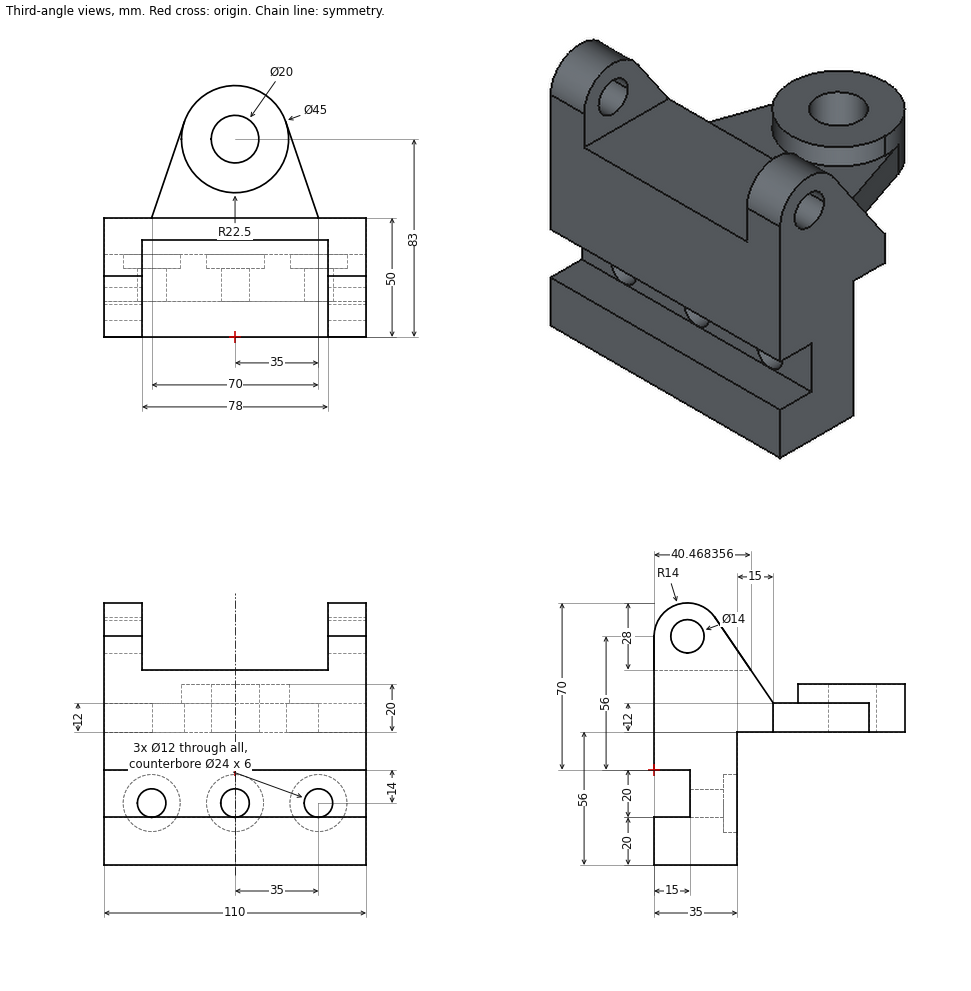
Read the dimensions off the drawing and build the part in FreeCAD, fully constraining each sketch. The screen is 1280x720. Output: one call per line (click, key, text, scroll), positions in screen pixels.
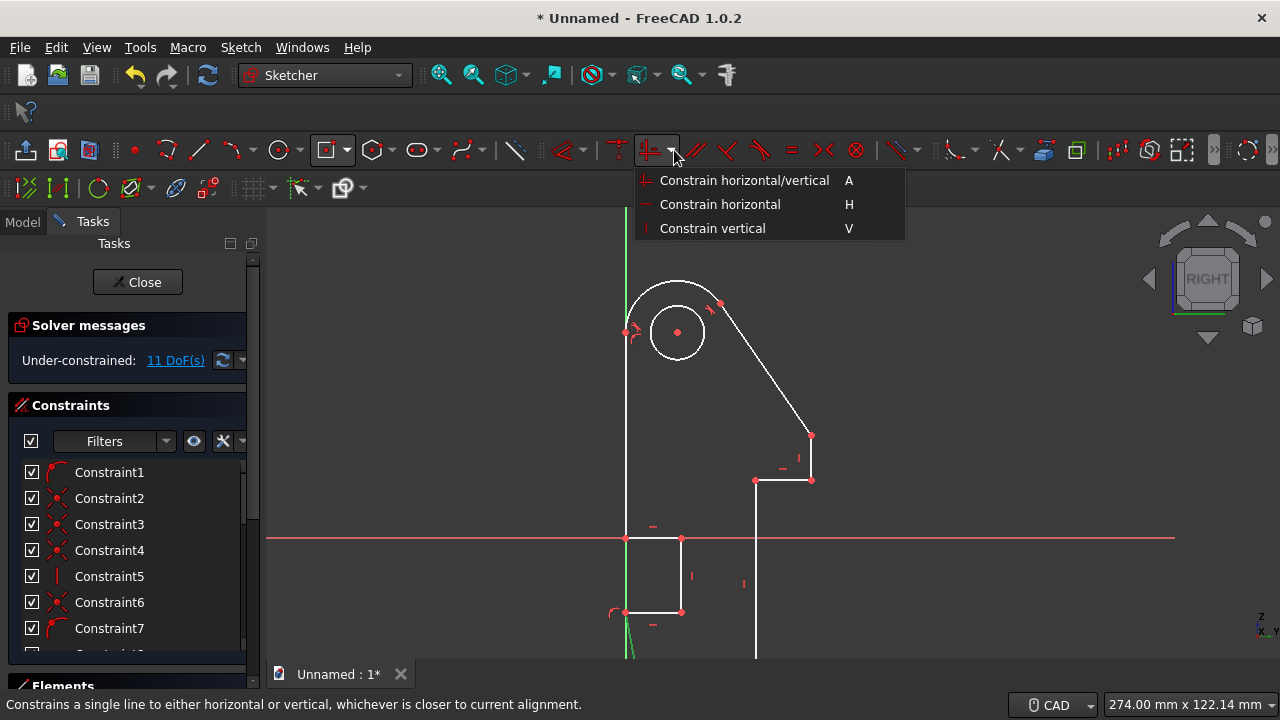
click(770, 228)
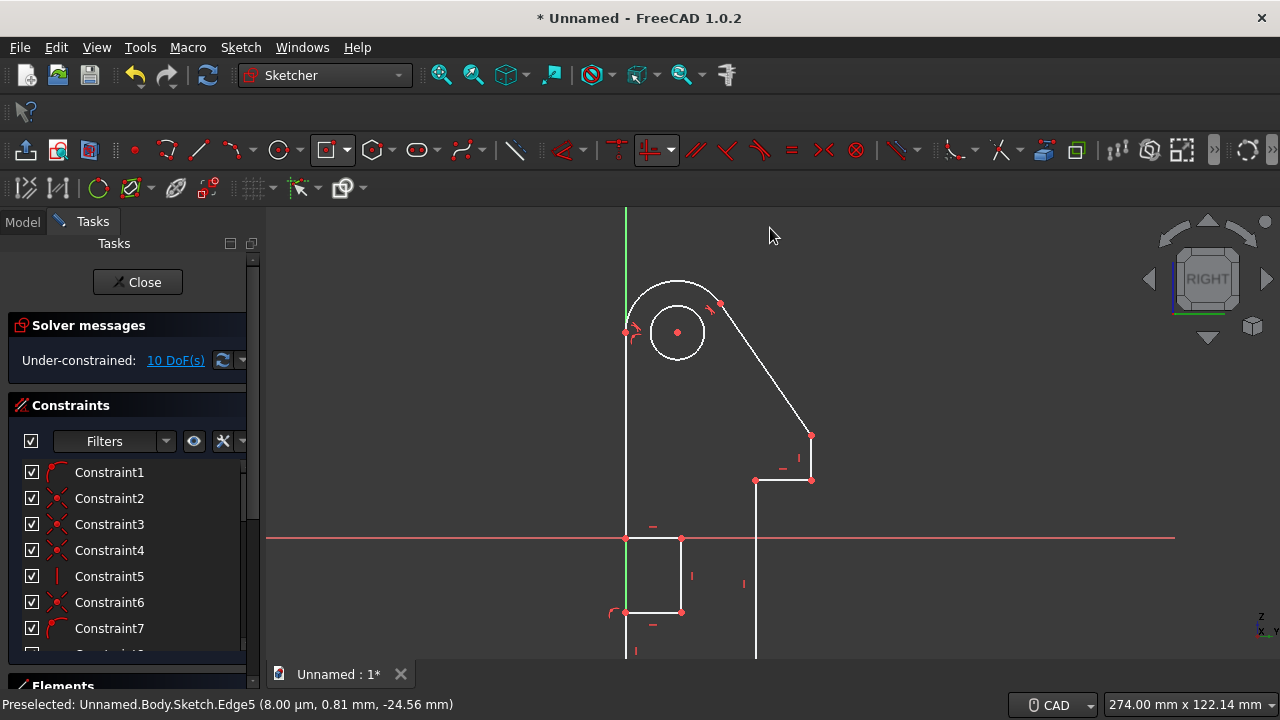
click(688, 282)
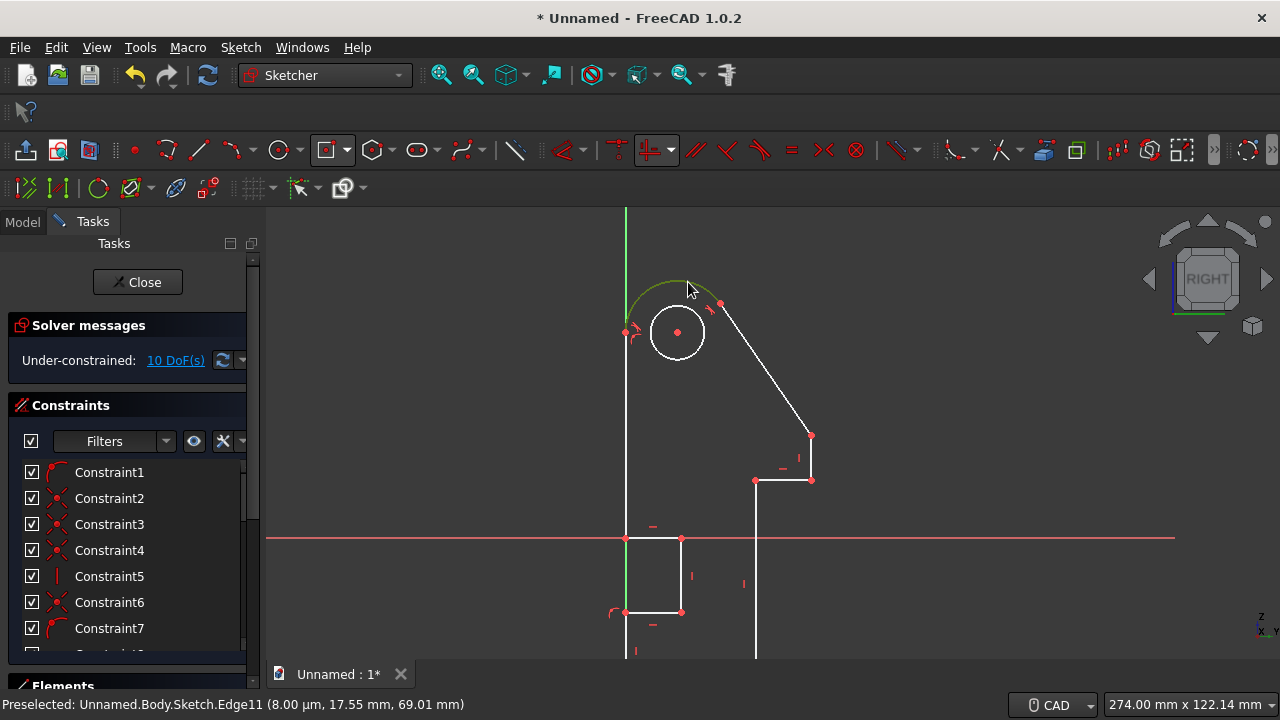
key(k)
key(r)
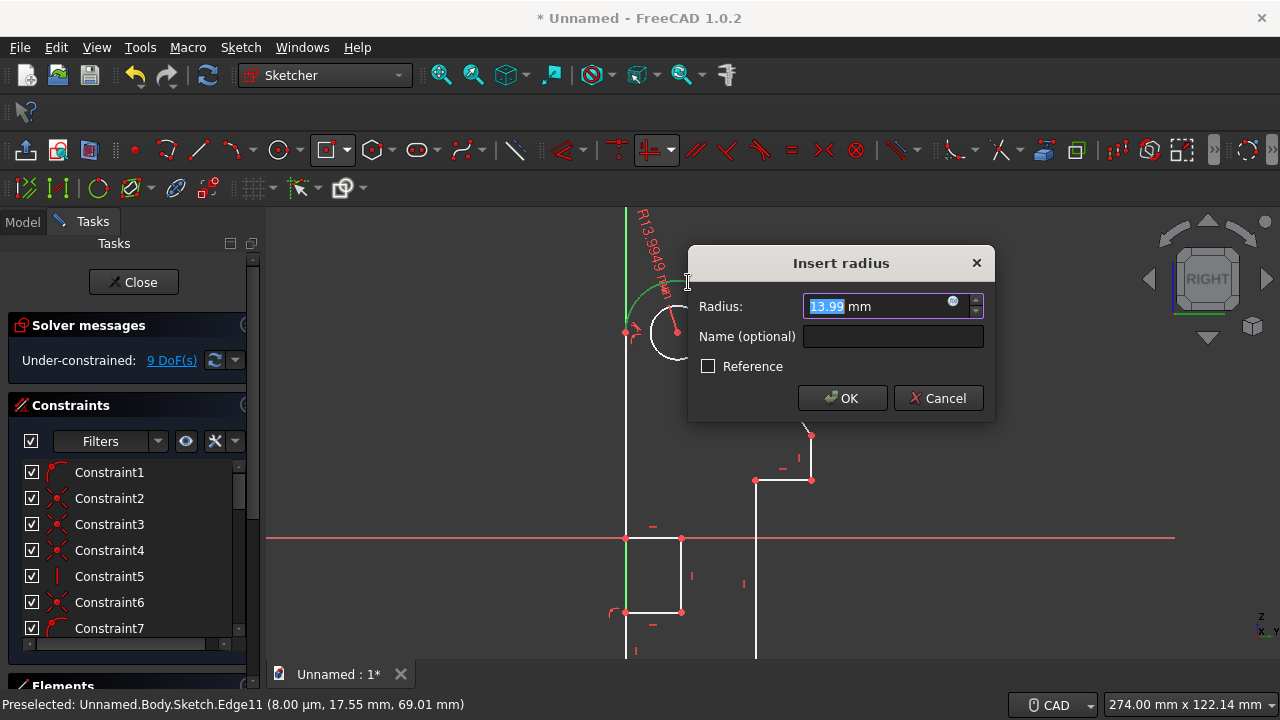
text(14)
key(Return)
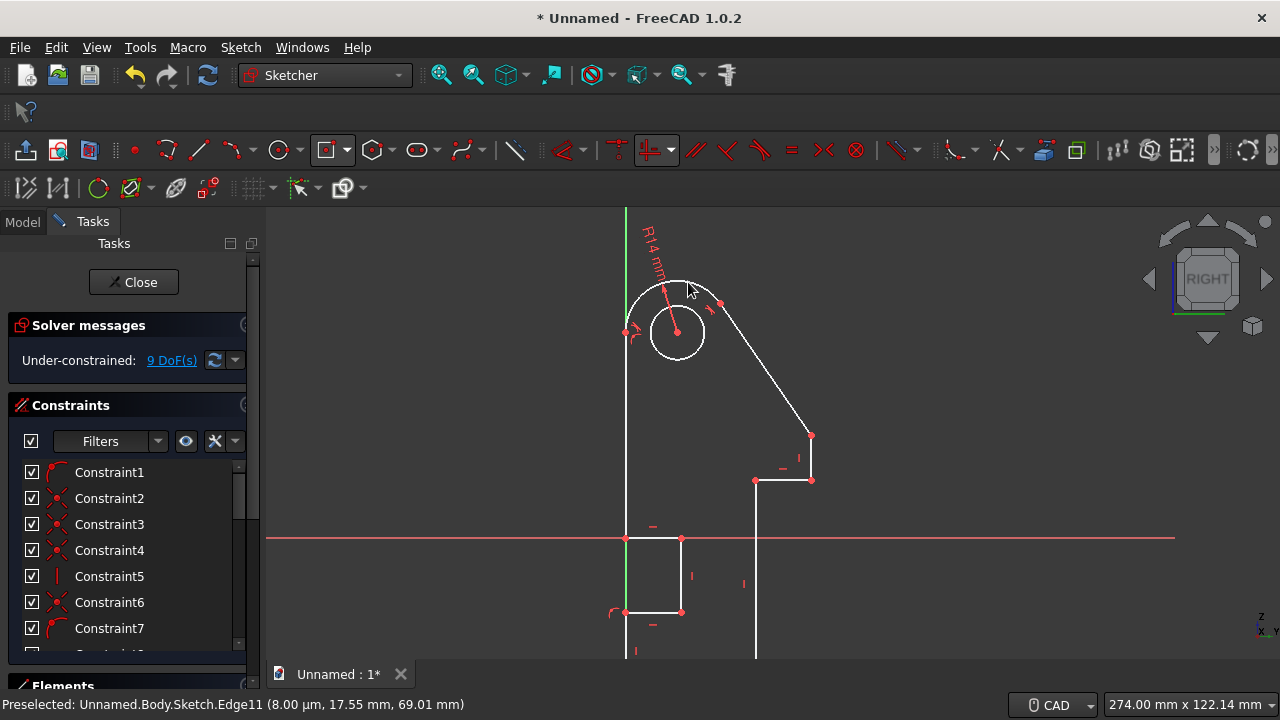
click(696, 314)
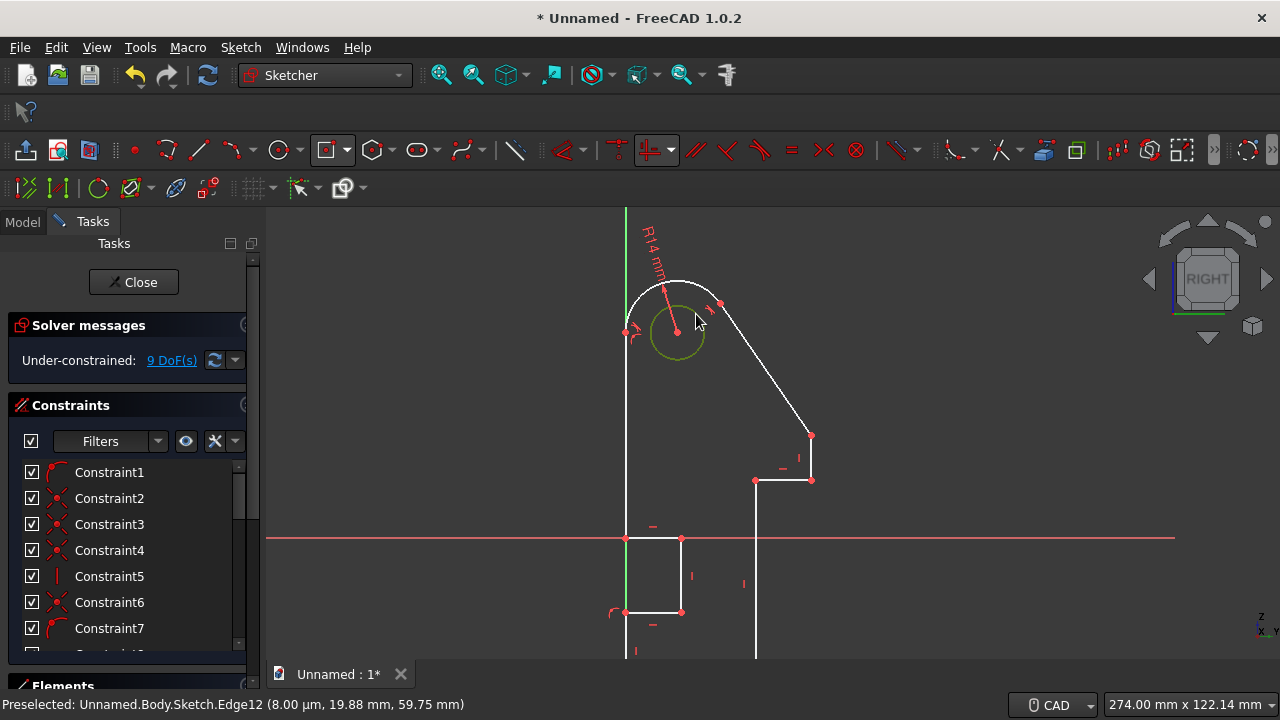
click(586, 150)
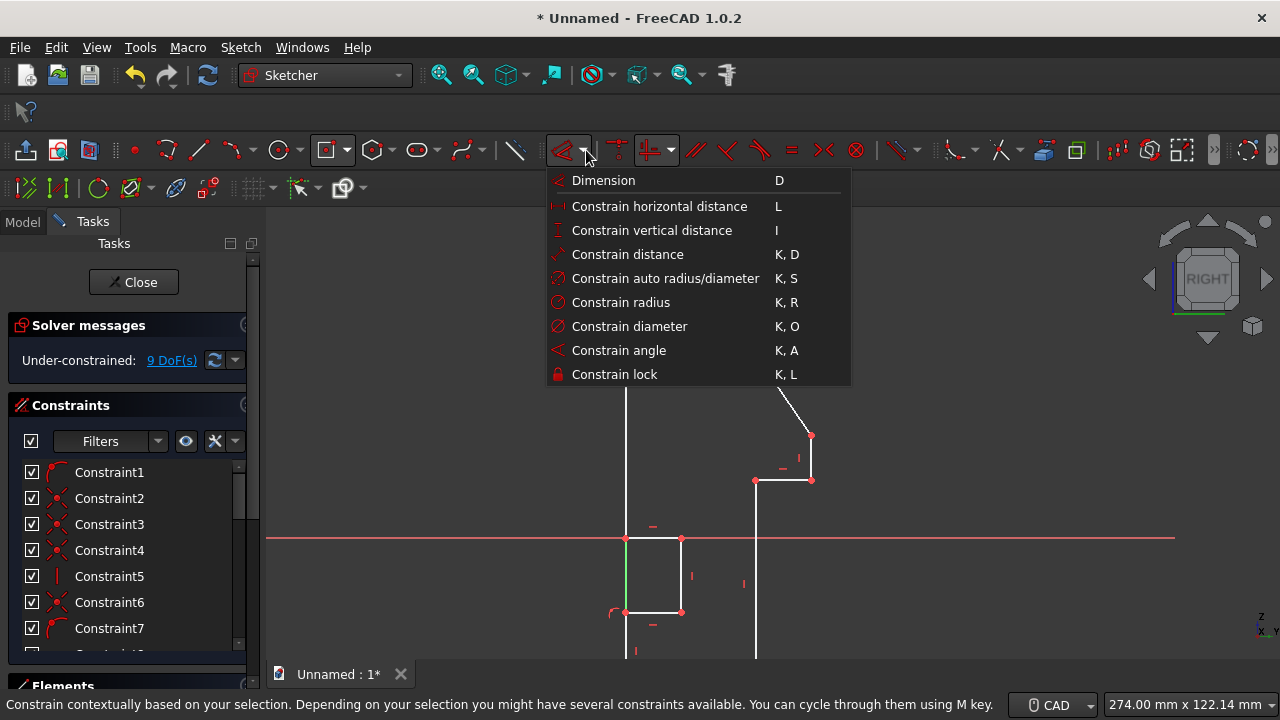
click(699, 326)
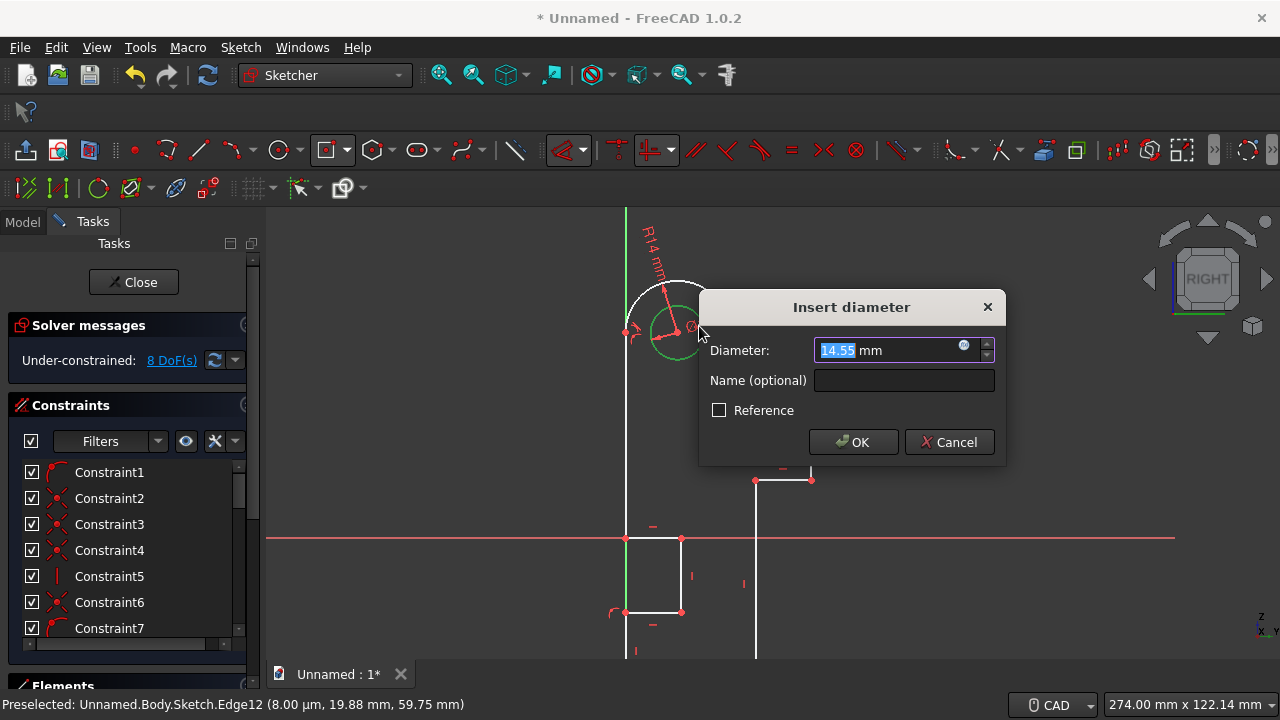
text(14)
key(Return)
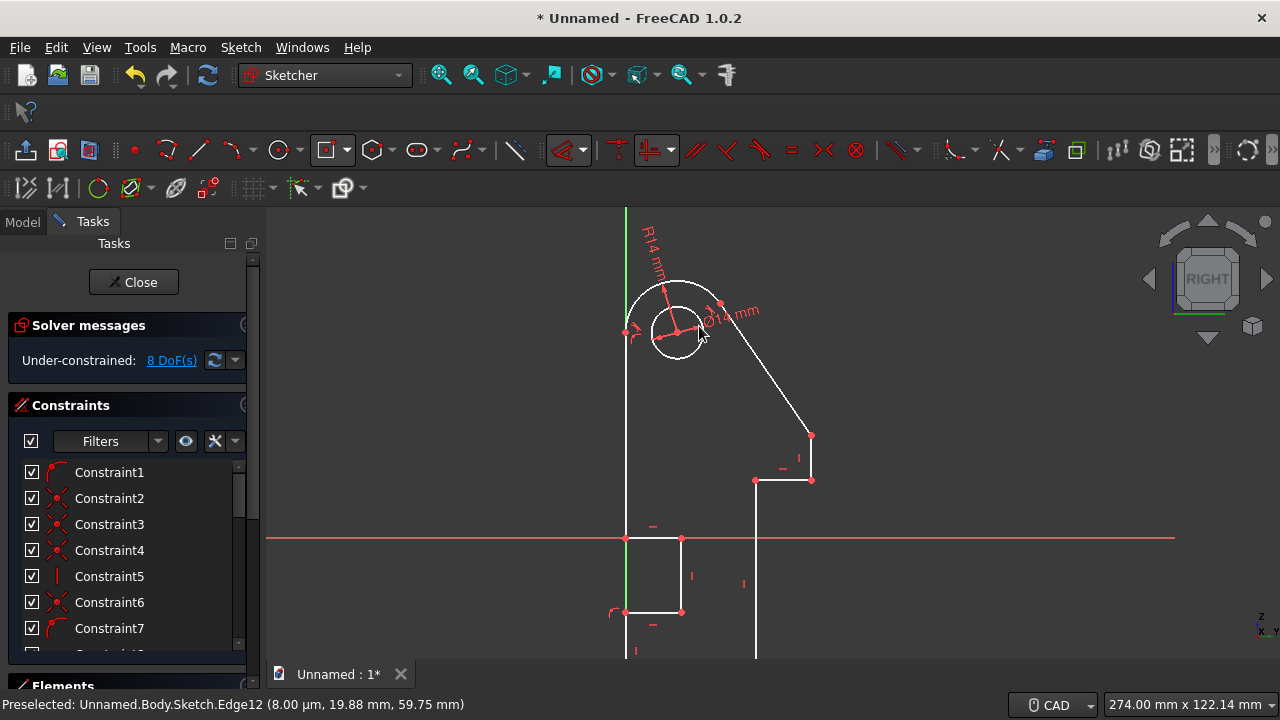
click(626, 394)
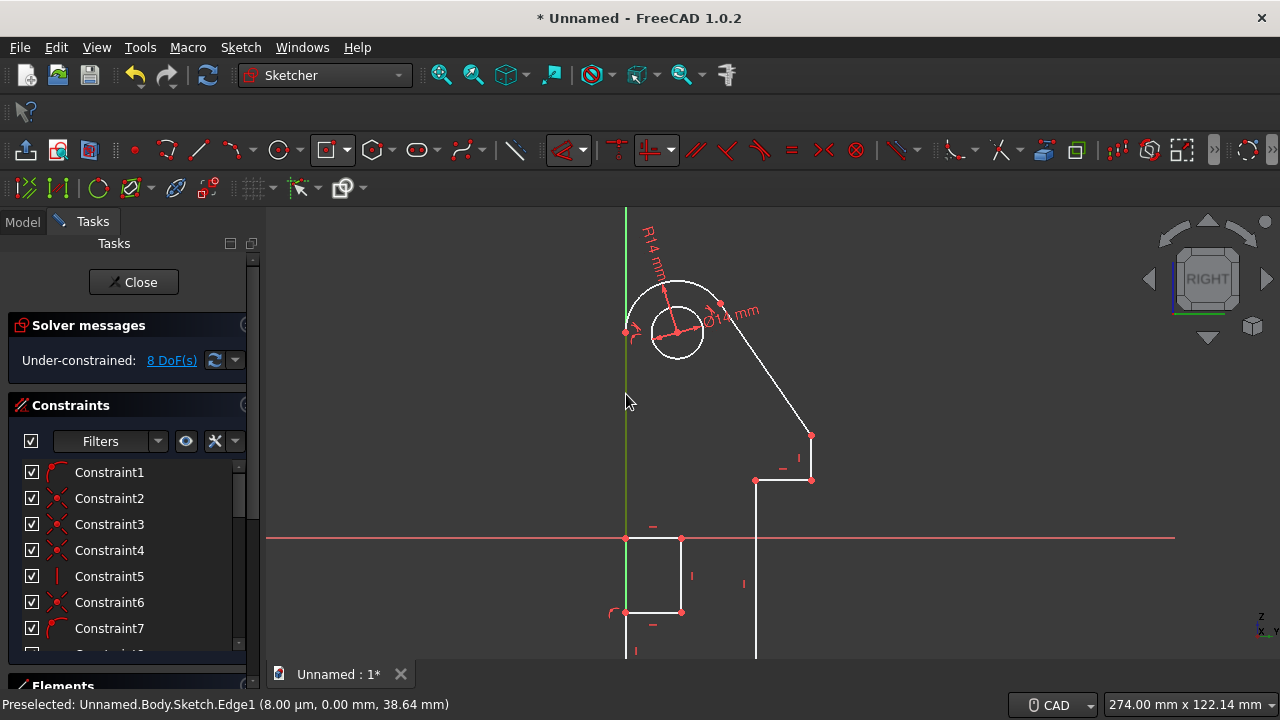
click(586, 150)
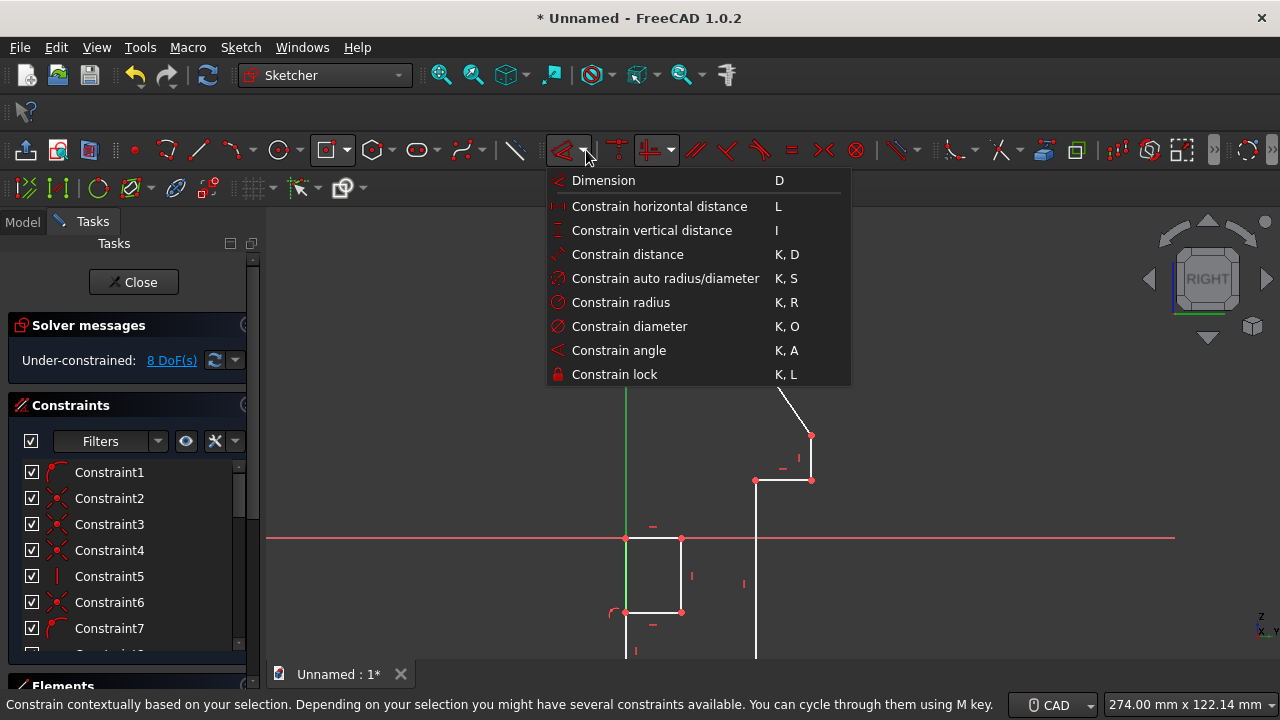
click(699, 230)